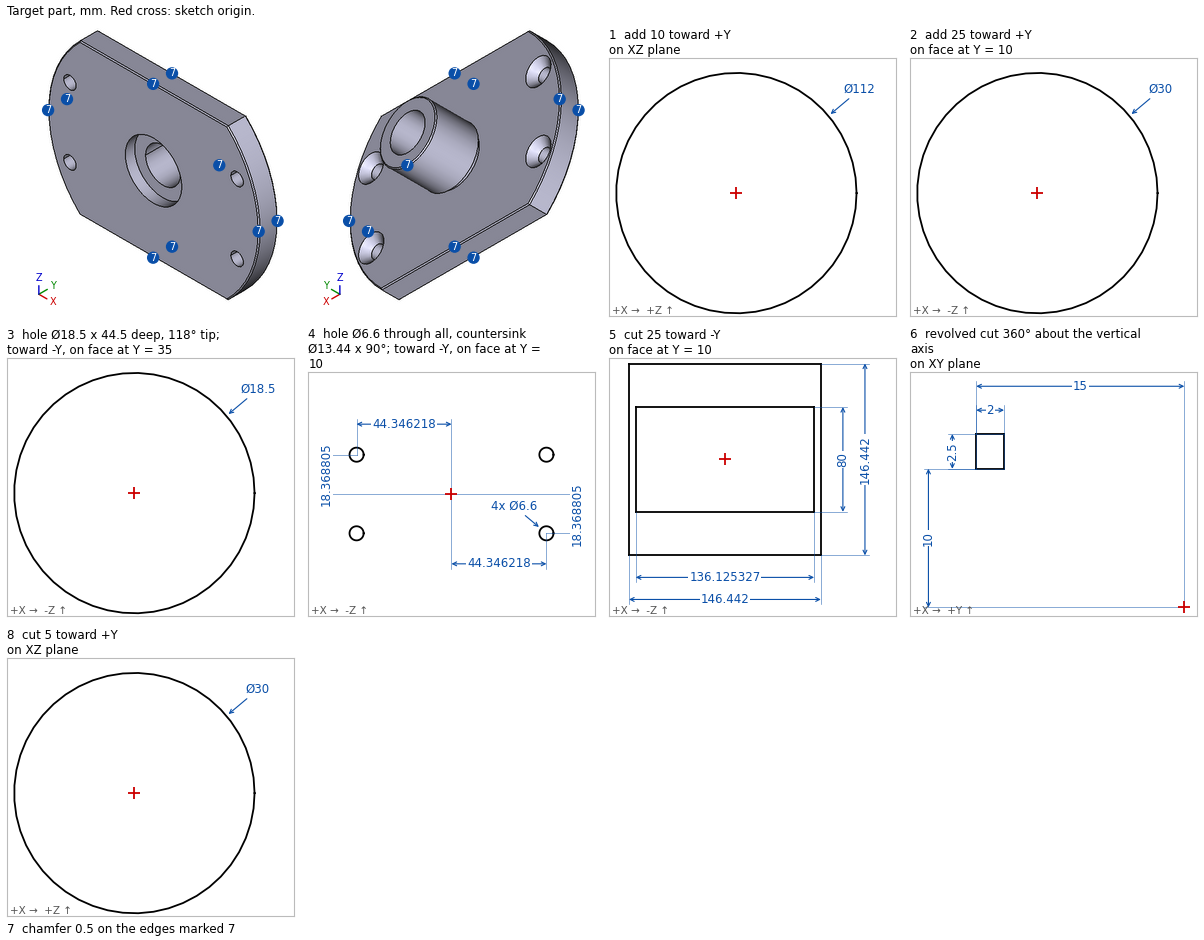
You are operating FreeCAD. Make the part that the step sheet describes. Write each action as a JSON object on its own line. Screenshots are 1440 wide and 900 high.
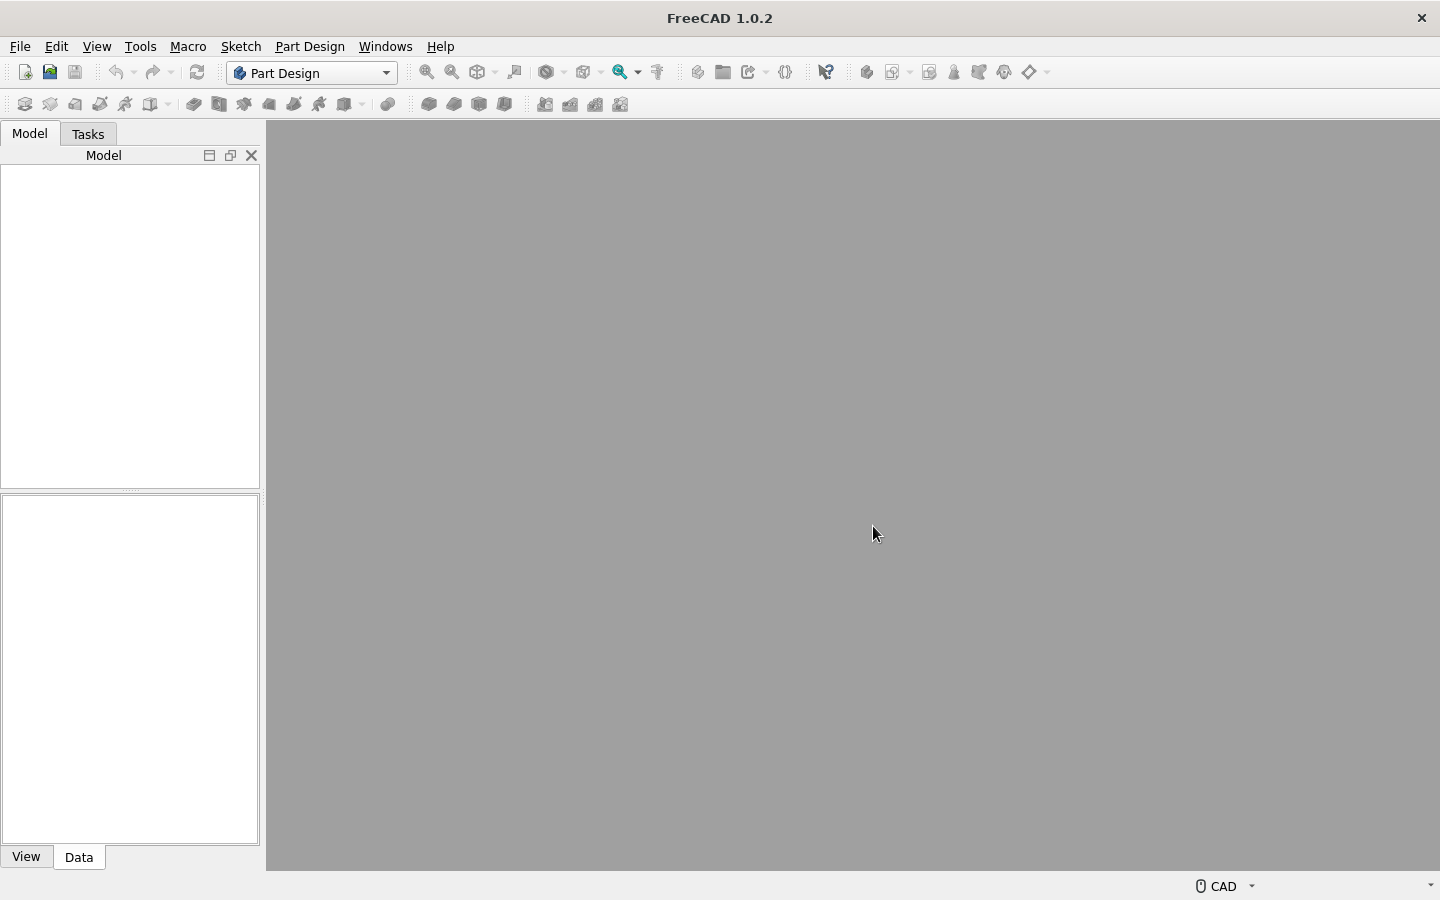
{"action": "left_click", "coordinate": [25, 72]}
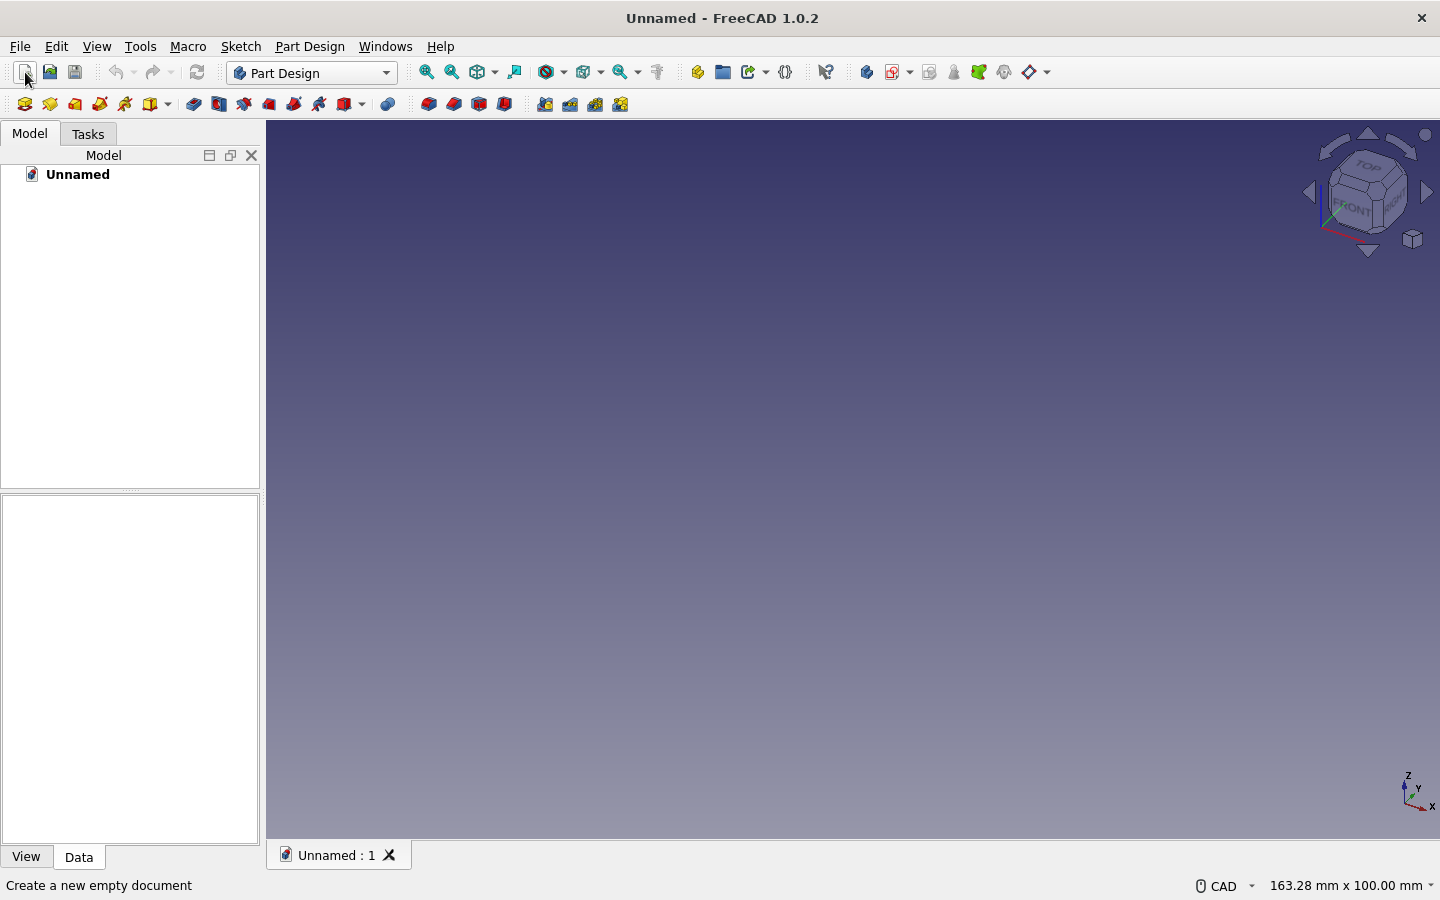
{"action": "left_click", "coordinate": [892, 72]}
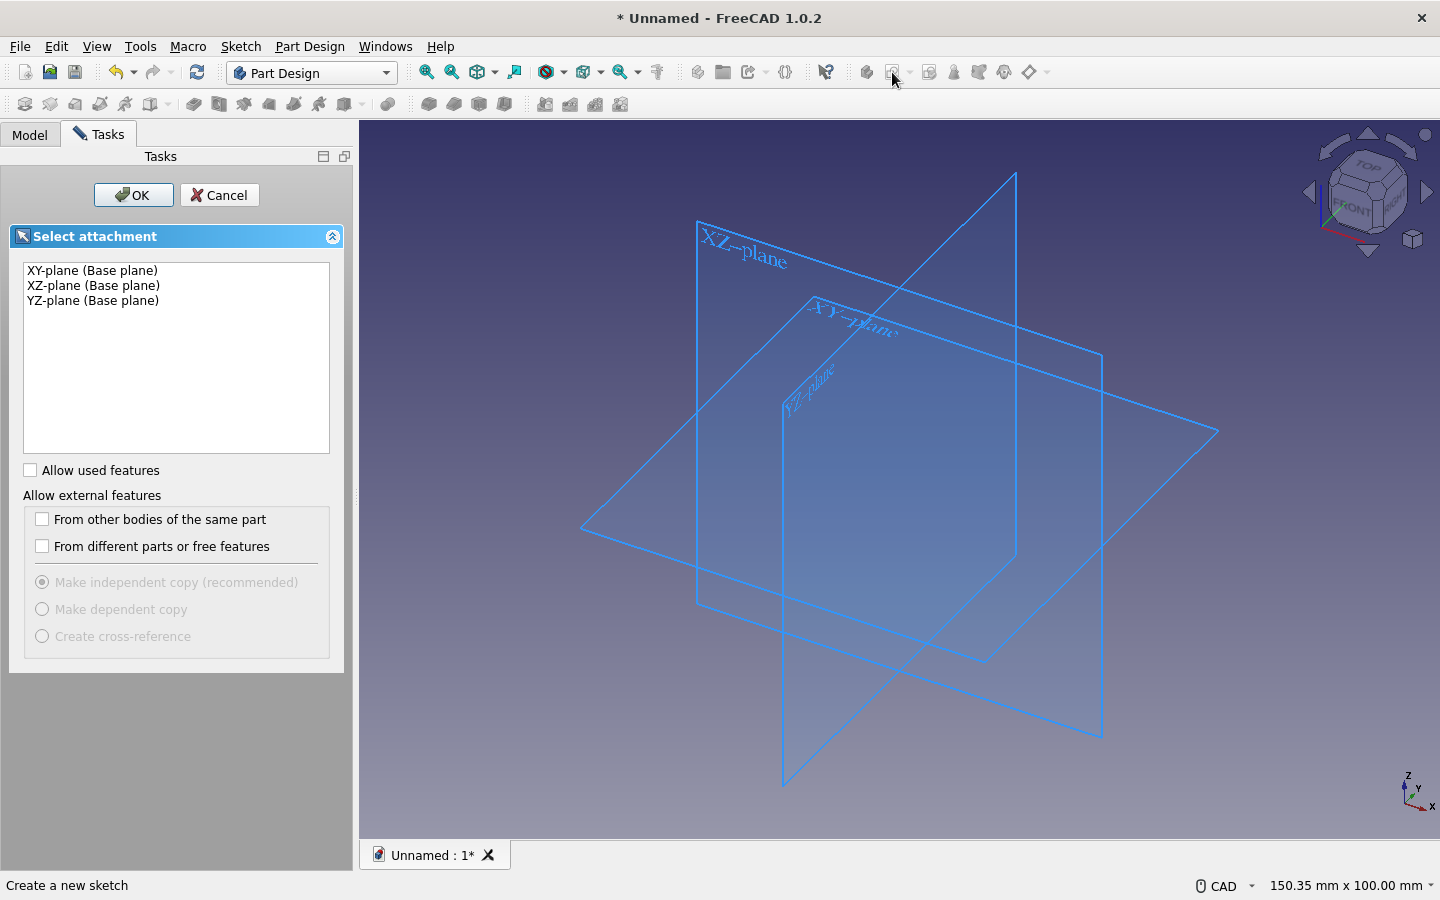
{"action": "left_click", "coordinate": [84, 286]}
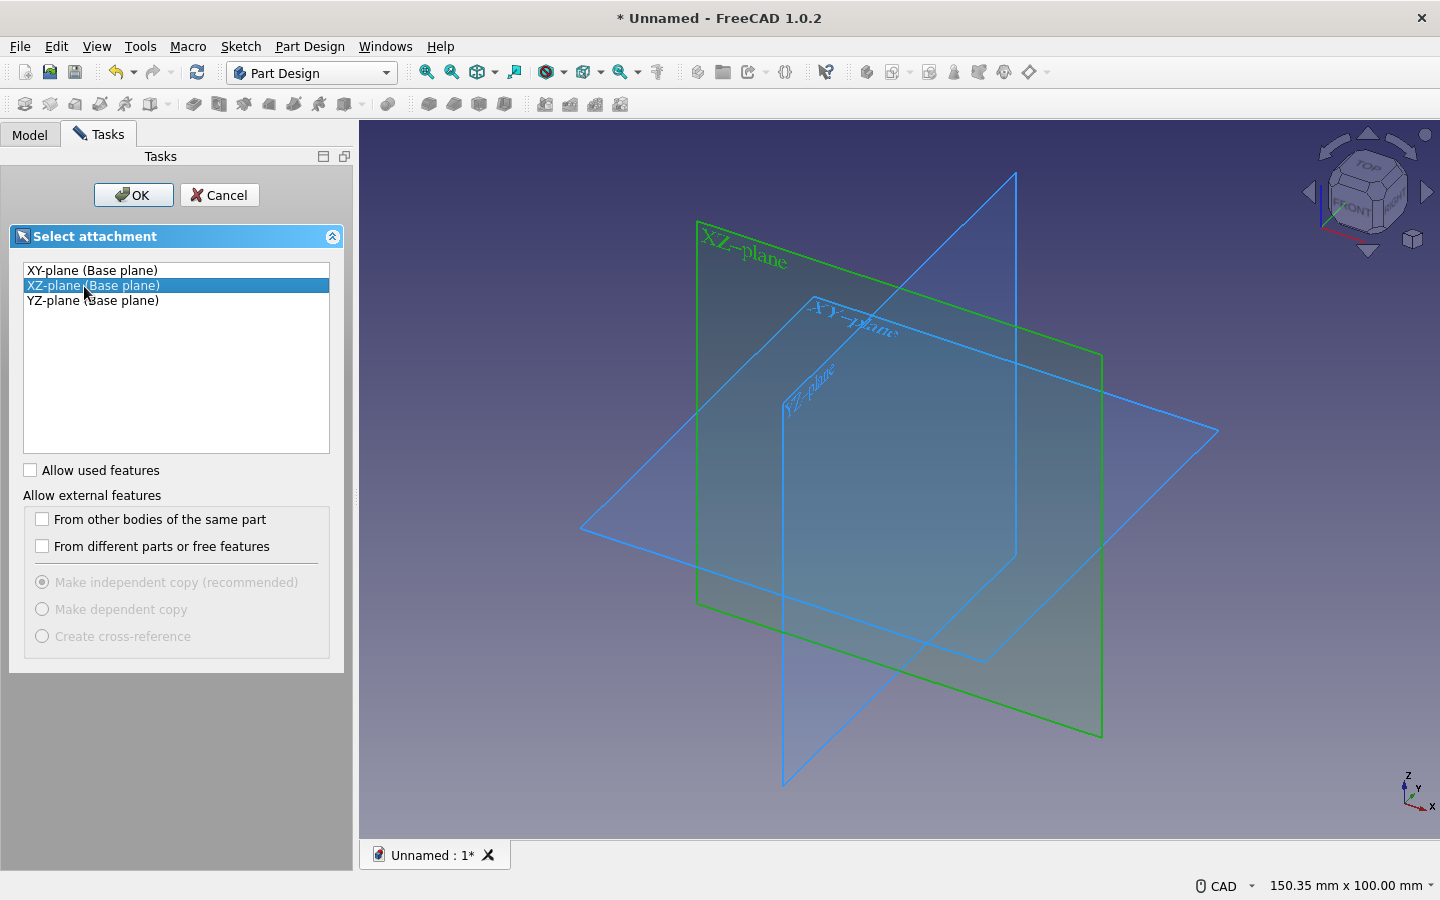
{"action": "left_click", "coordinate": [134, 195]}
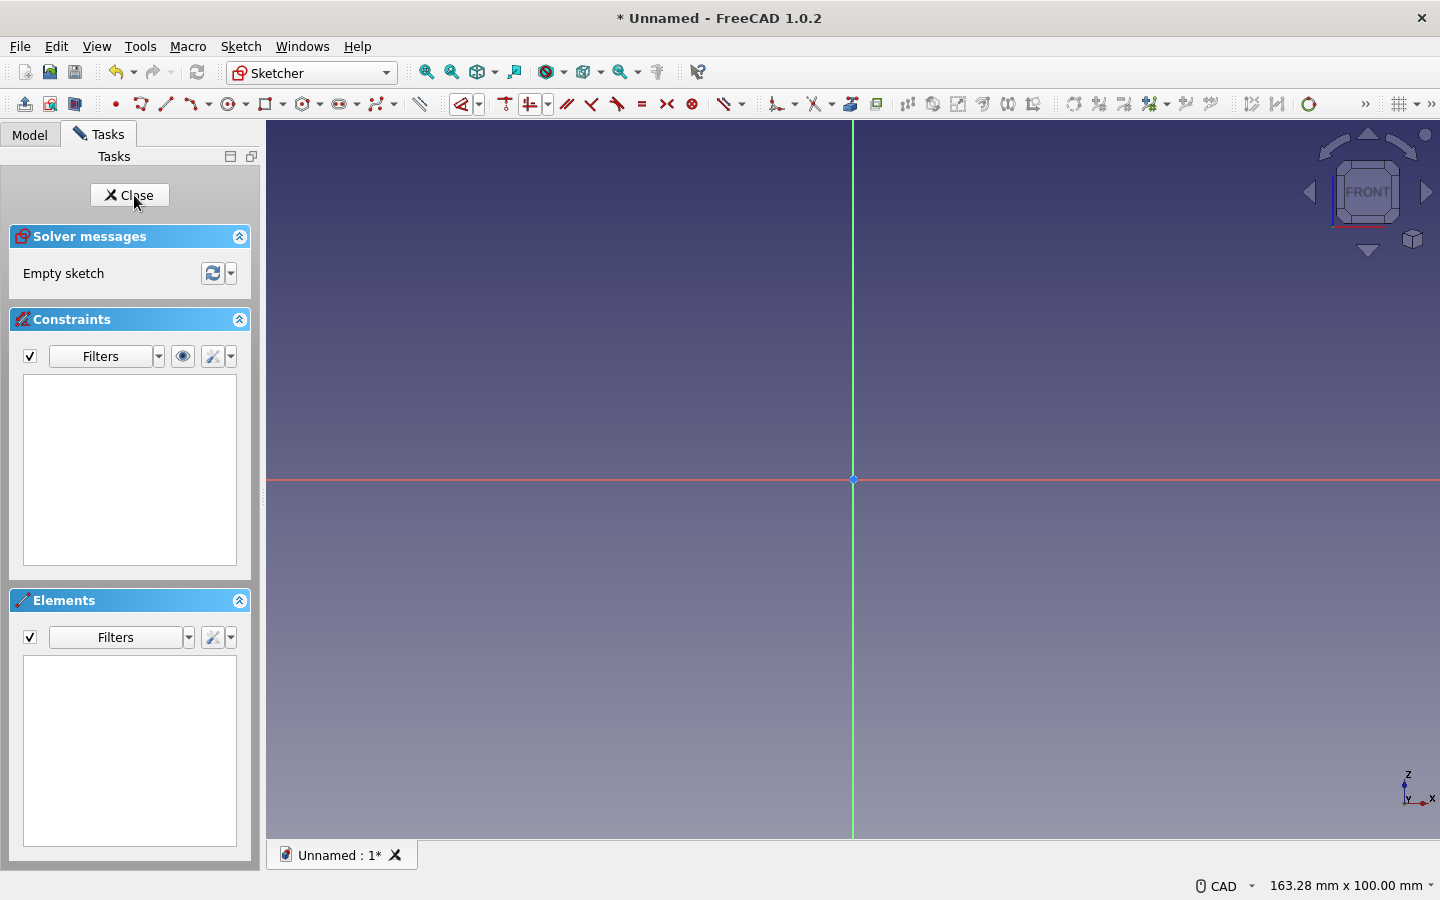
{"action": "scroll", "coordinate": [701, 479], "scroll_direction": "down", "scroll_amount": 3}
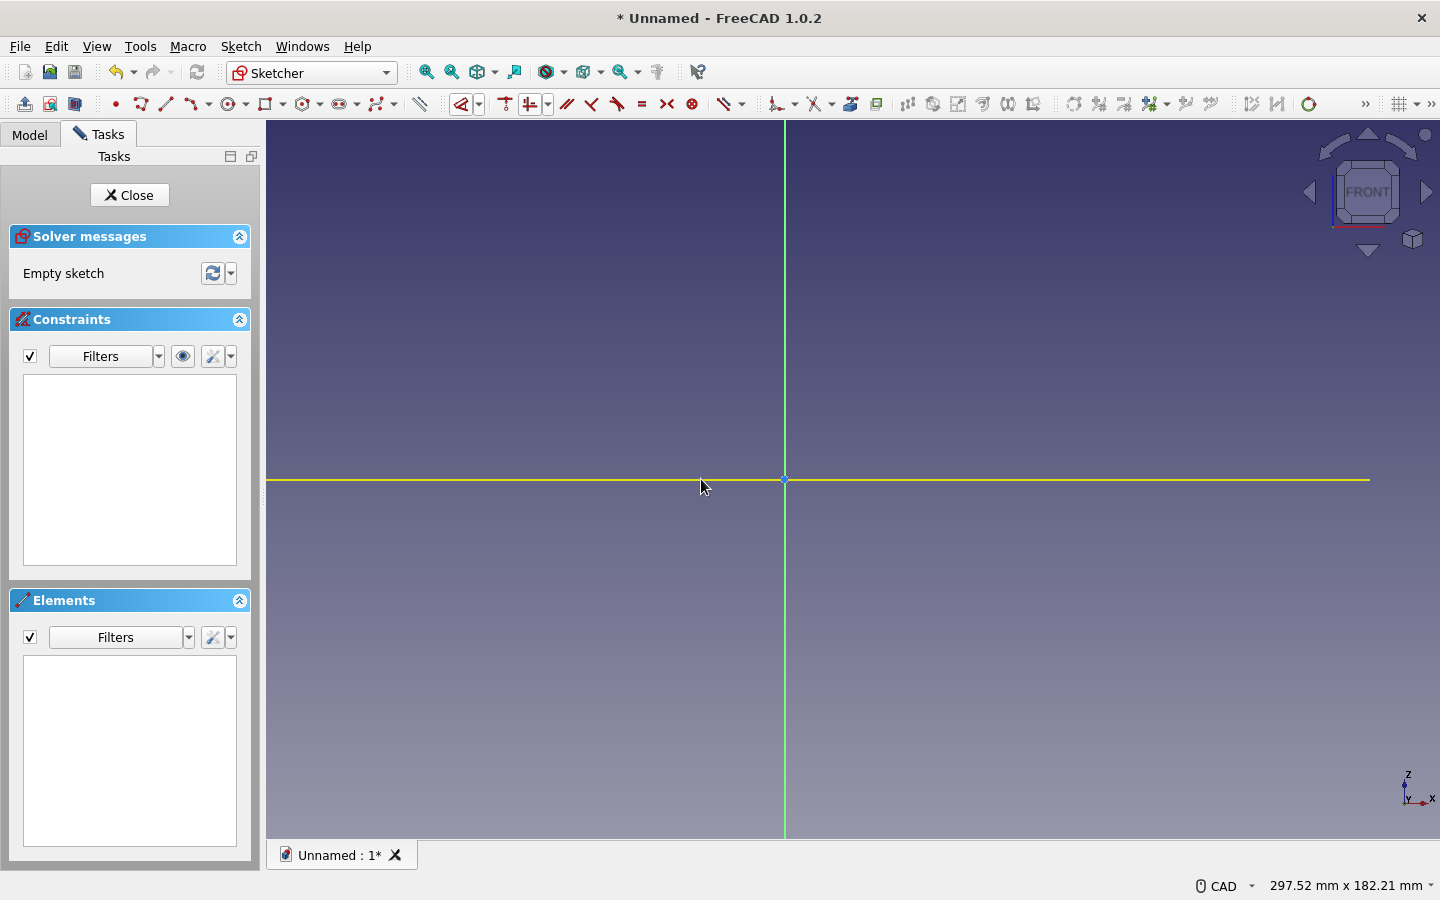
{"action": "key", "text": "g c"}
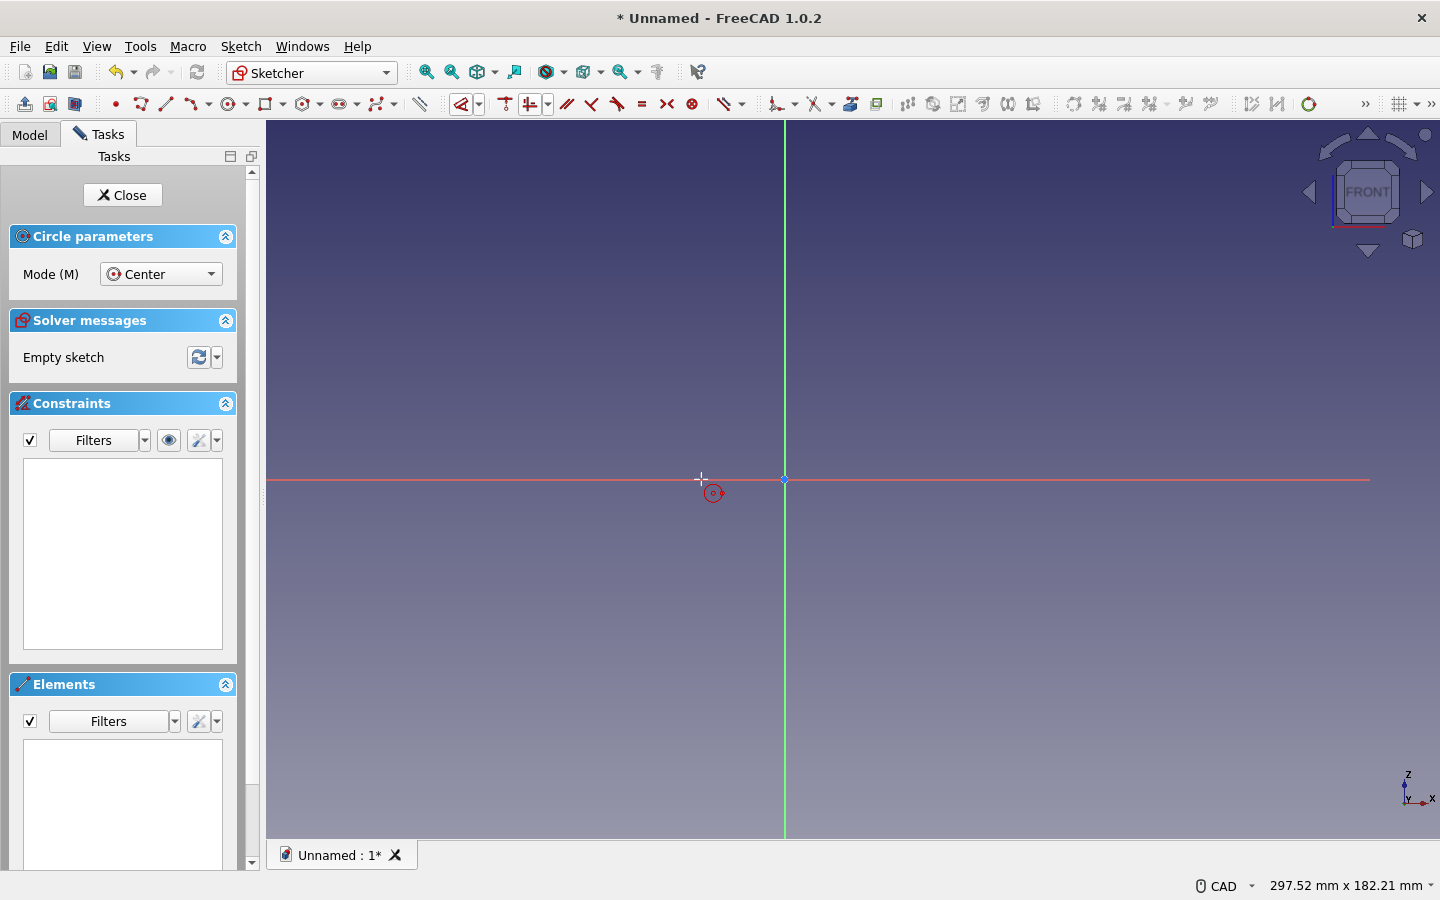
{"action": "left_click", "coordinate": [785, 480]}
{"action": "mouse_move", "coordinate": [941, 323]}